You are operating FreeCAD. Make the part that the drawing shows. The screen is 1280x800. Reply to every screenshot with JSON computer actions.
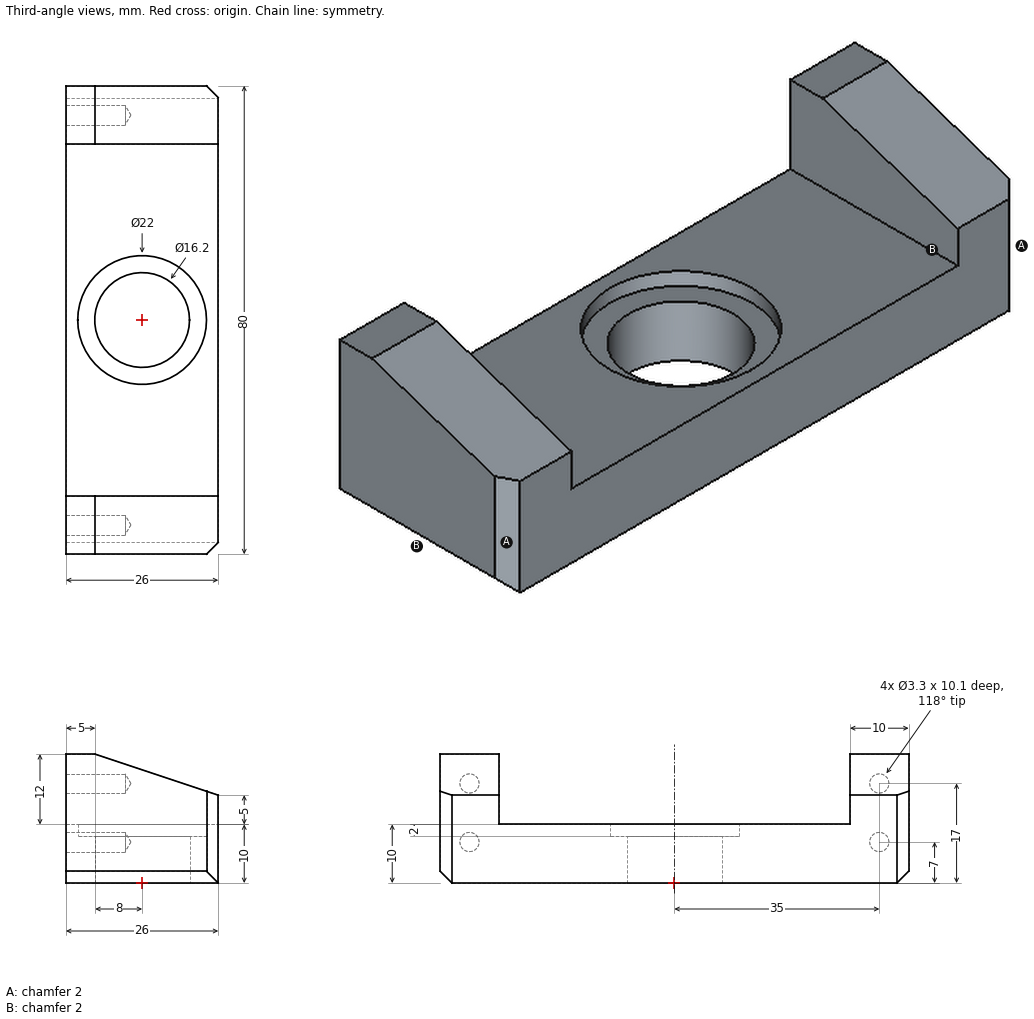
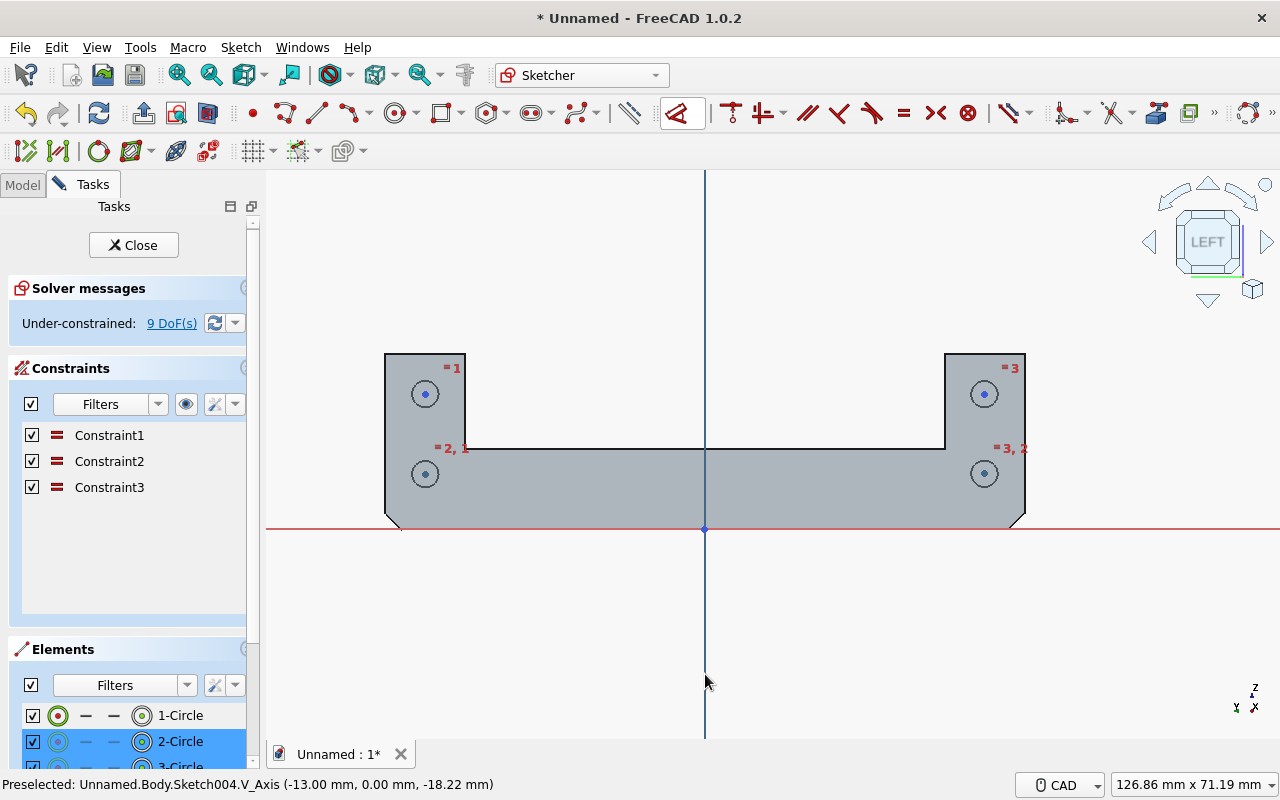
{"action": "key", "text": "s"}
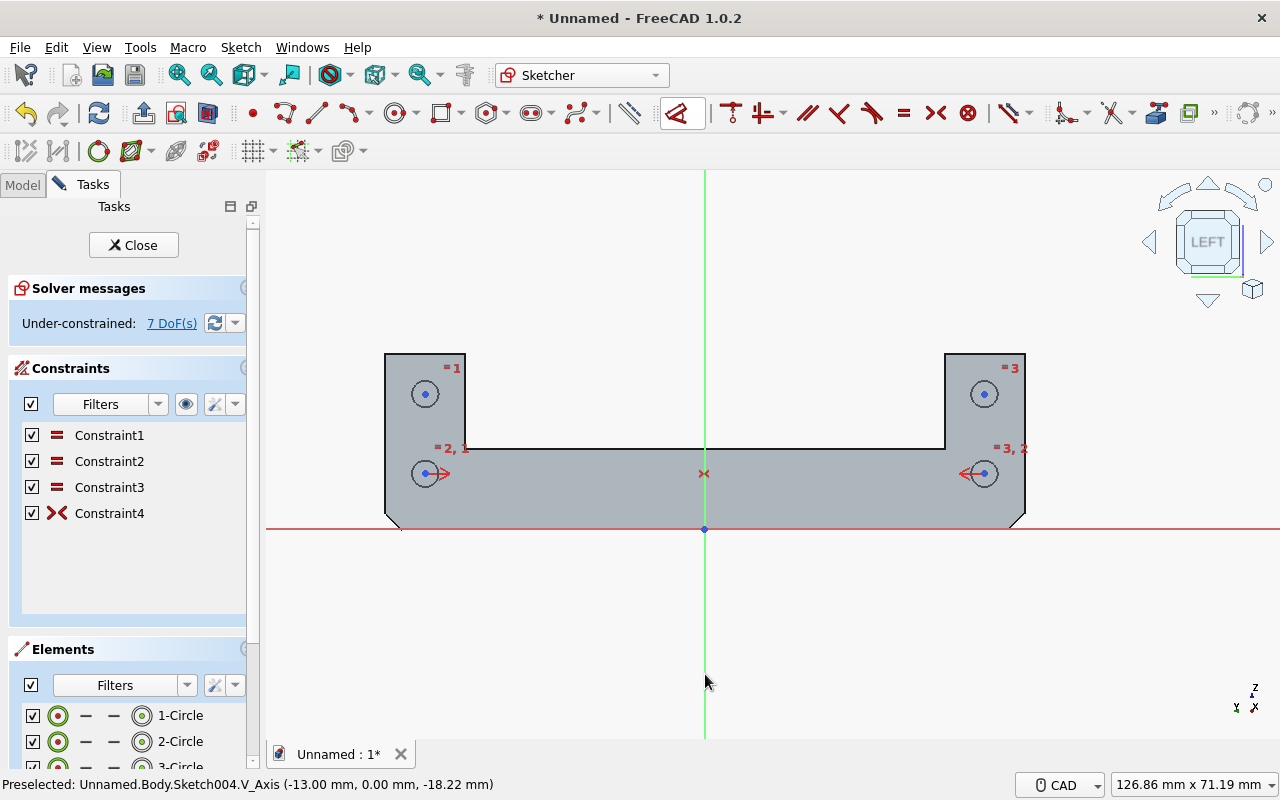
{"action": "left_click", "coordinate": [425, 394]}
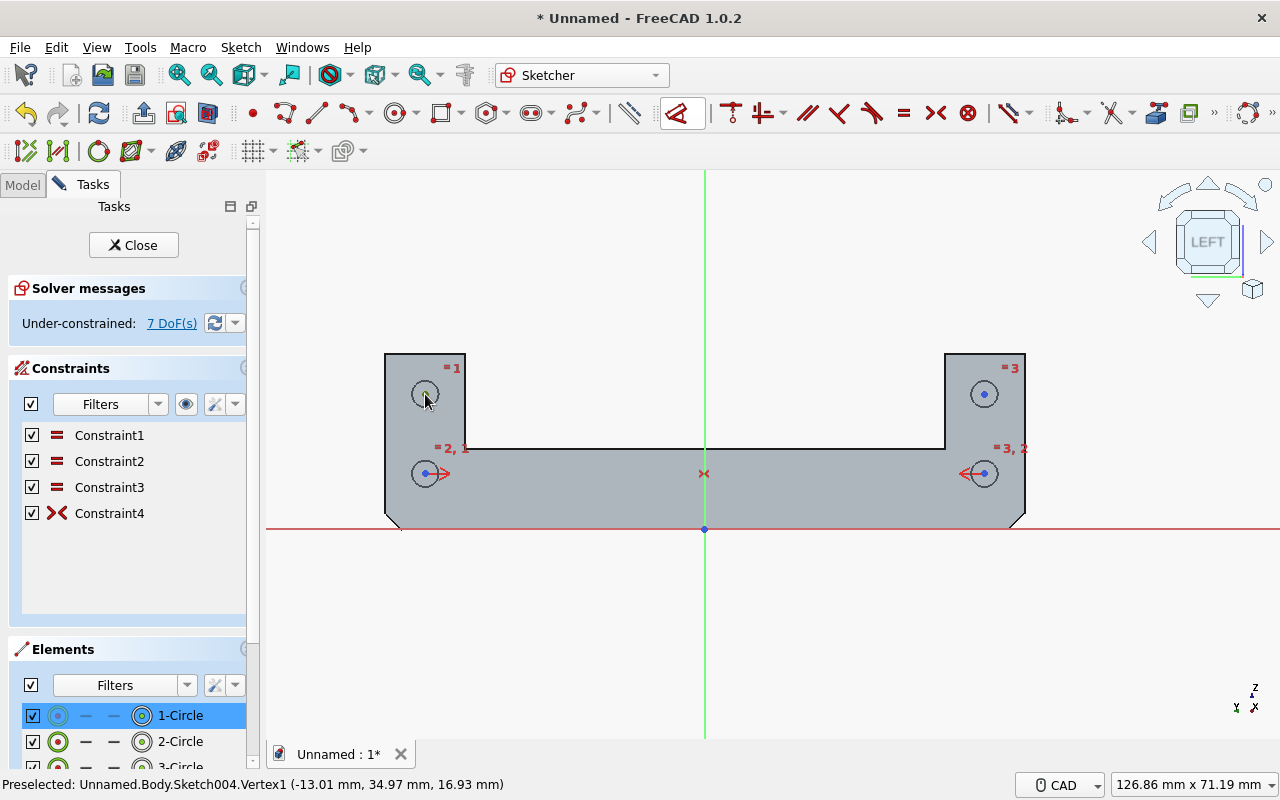
{"action": "left_click", "coordinate": [984, 394]}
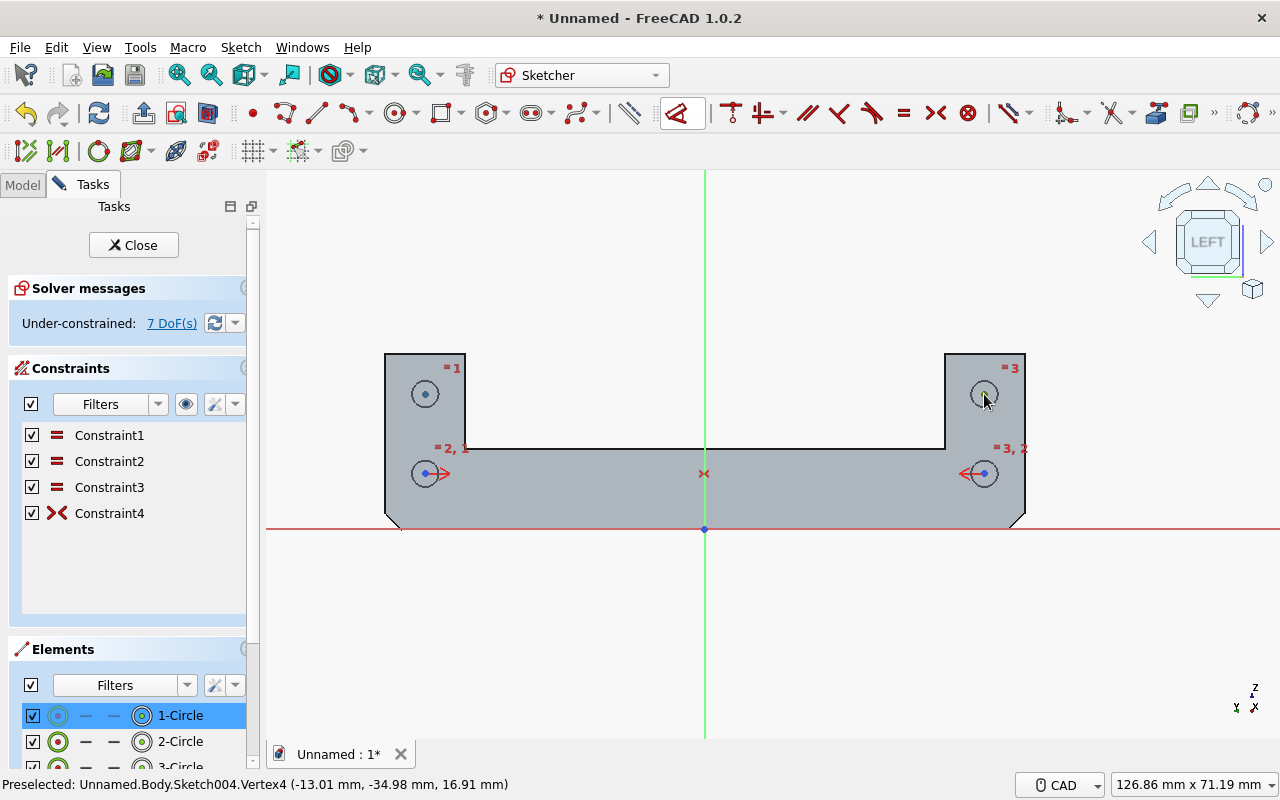
{"action": "left_click", "coordinate": [705, 674]}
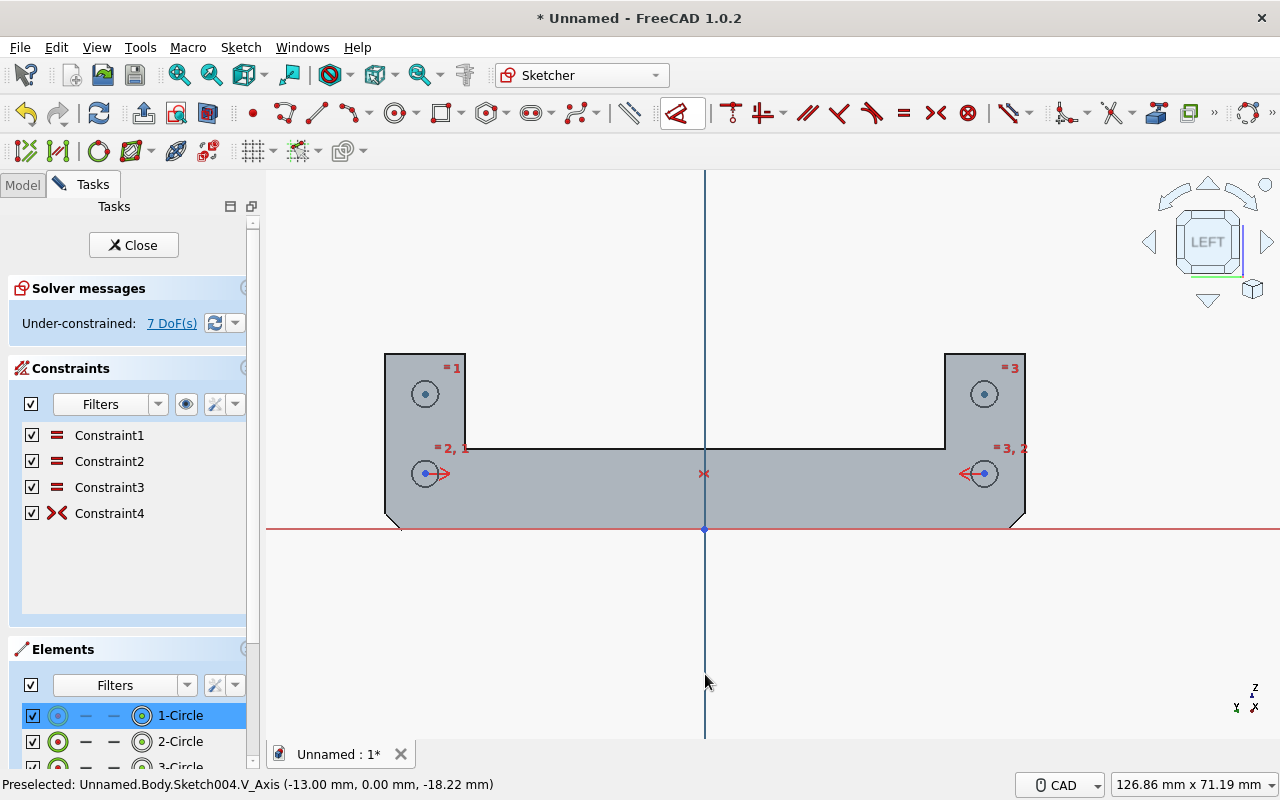
{"action": "left_click", "coordinate": [936, 114]}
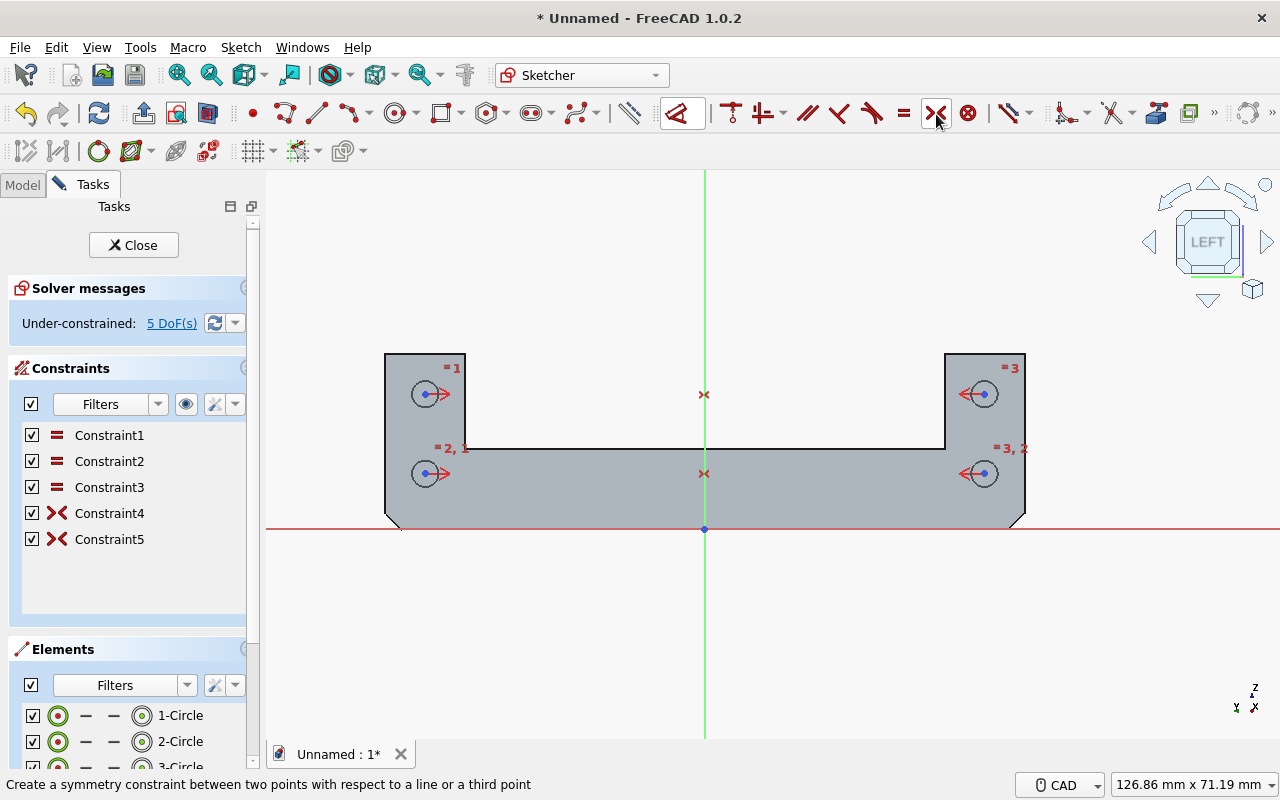
{"action": "scroll", "coordinate": [435, 385], "scroll_direction": "up", "scroll_amount": 3}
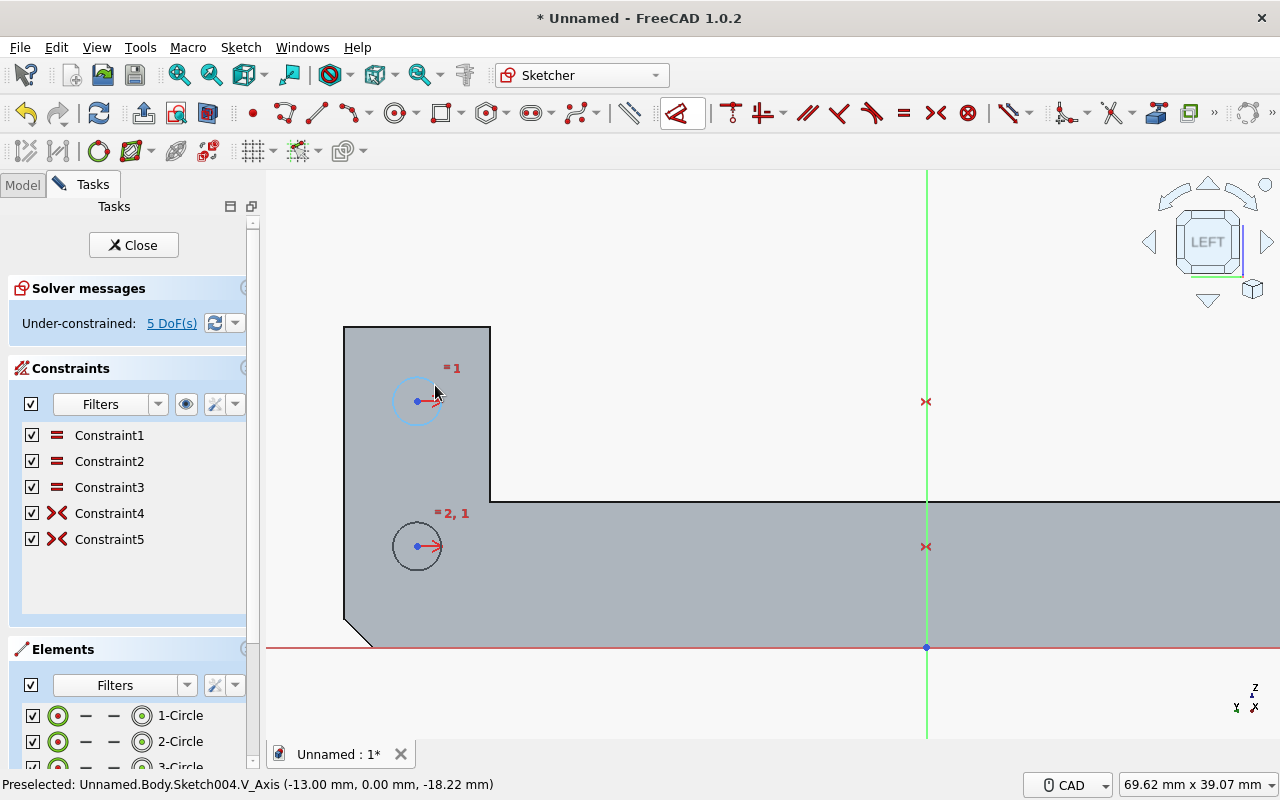
{"action": "left_click", "coordinate": [434, 384]}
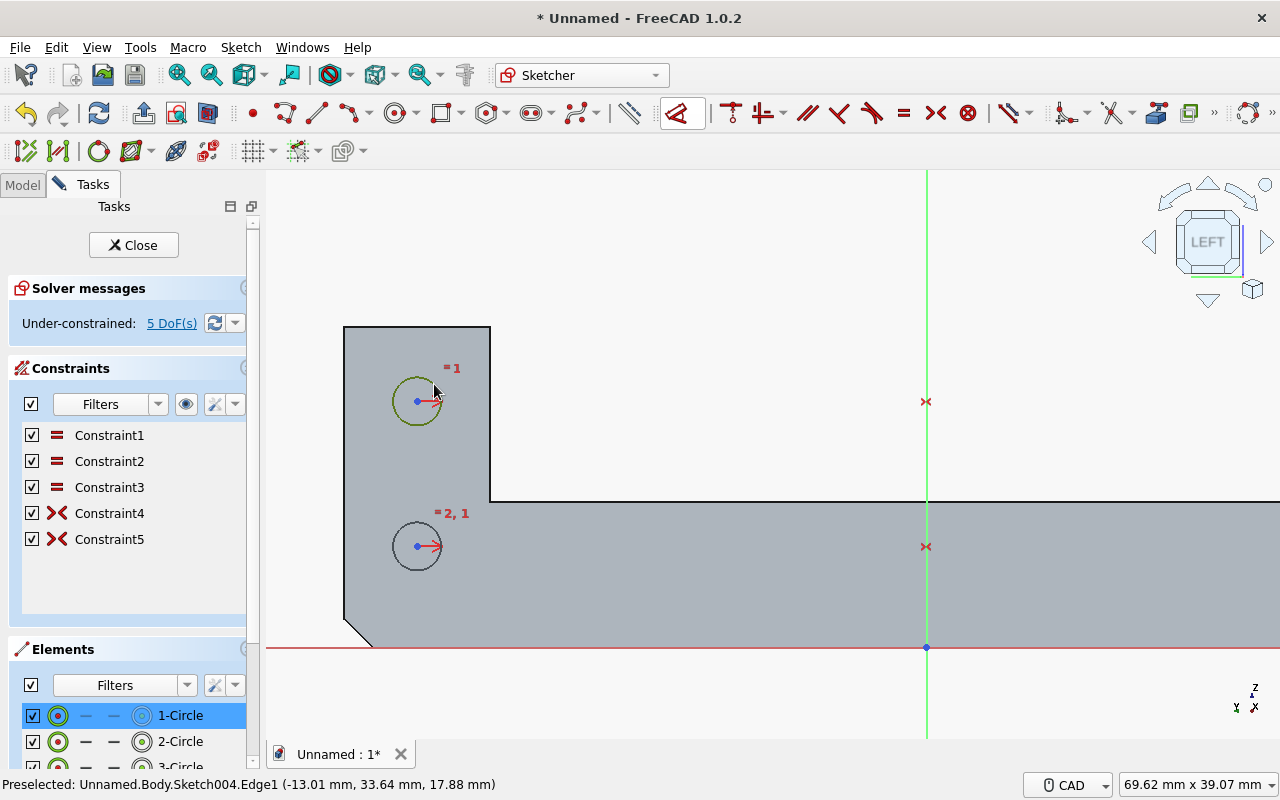
{"action": "left_click", "coordinate": [700, 114]}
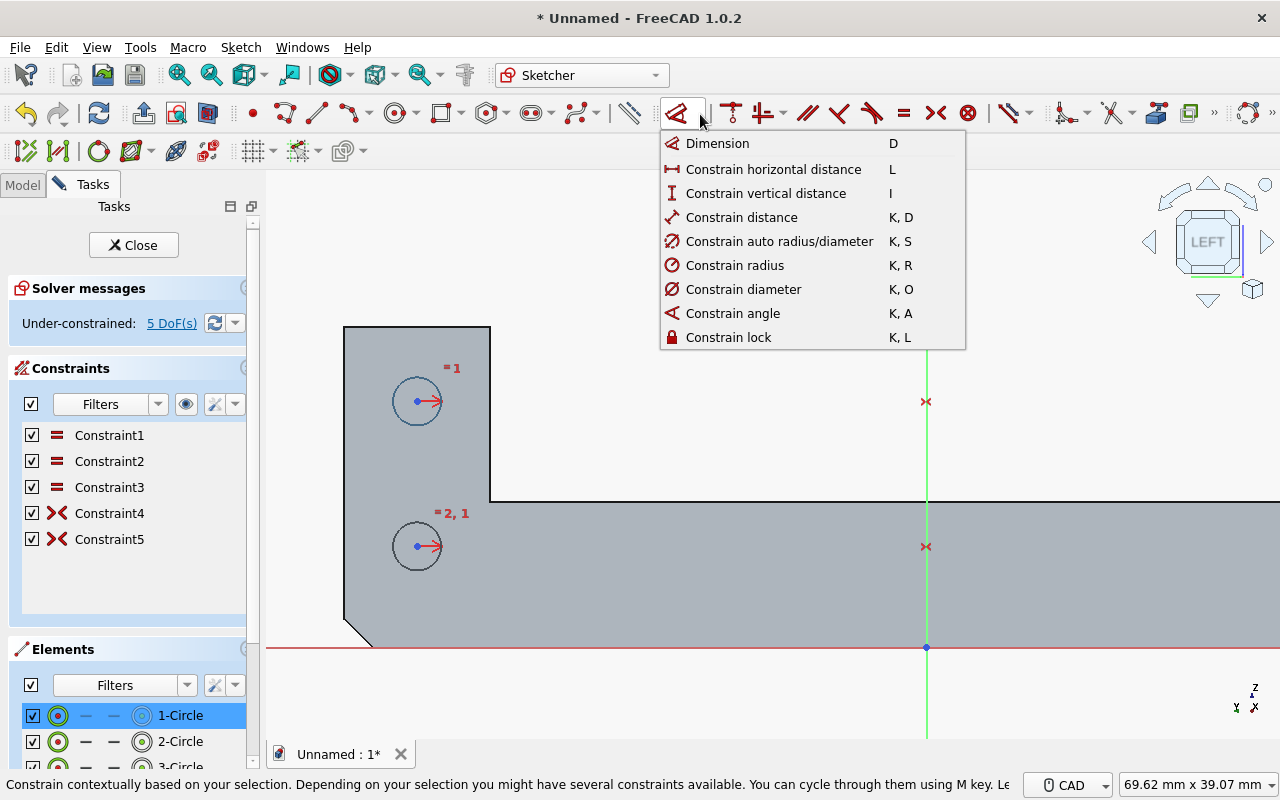
{"action": "left_click", "coordinate": [813, 289]}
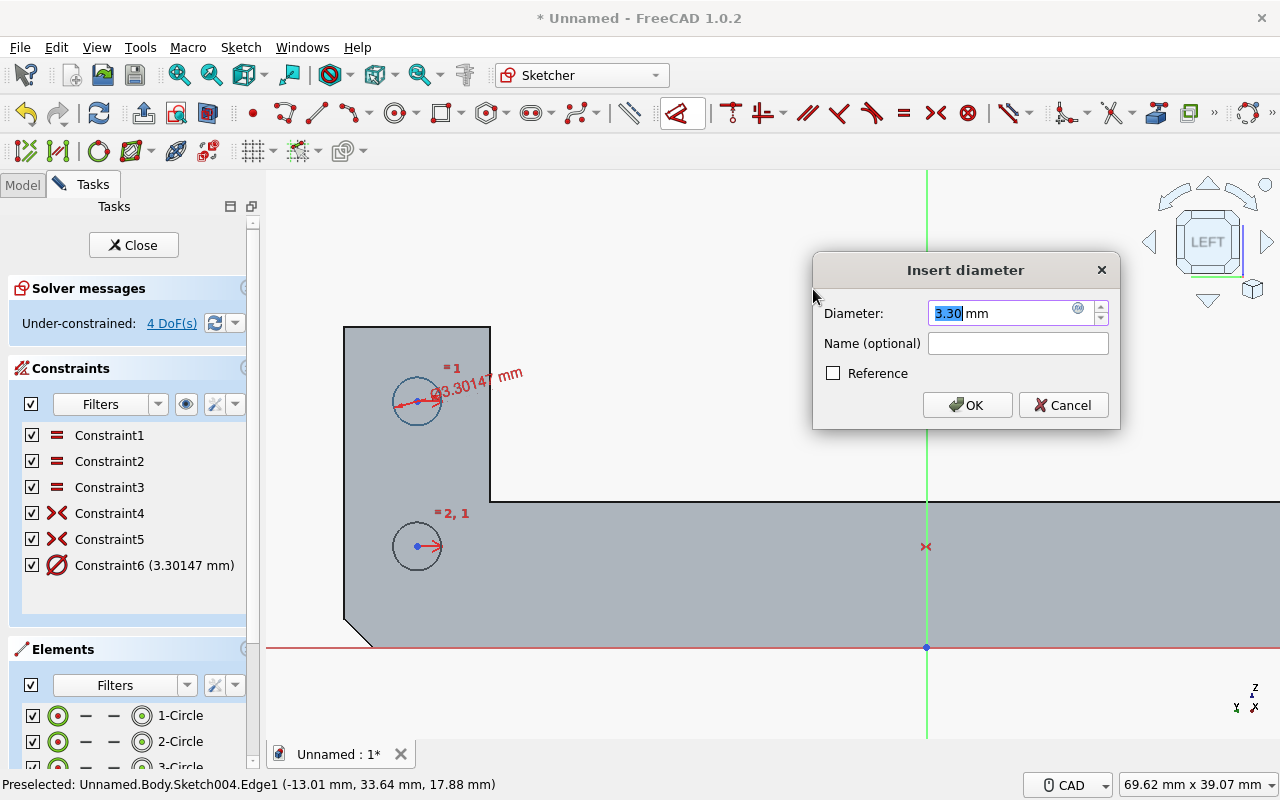
{"action": "type", "text": "3.3"}
{"action": "key", "text": "Return"}